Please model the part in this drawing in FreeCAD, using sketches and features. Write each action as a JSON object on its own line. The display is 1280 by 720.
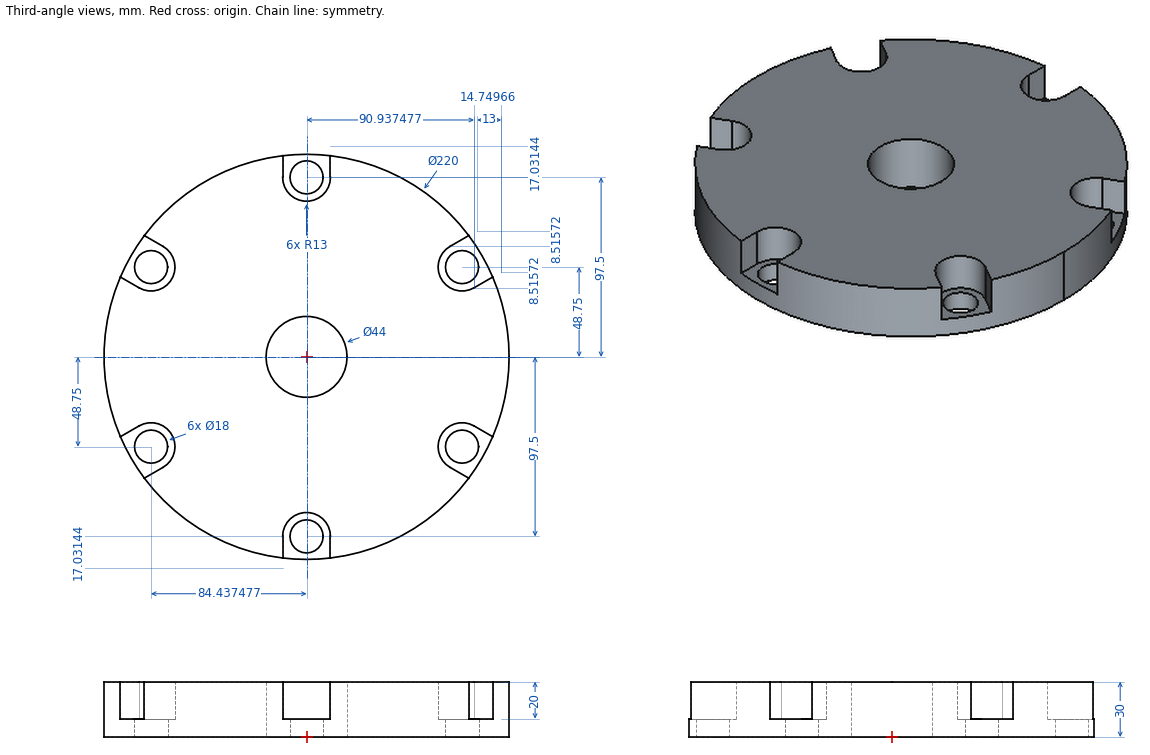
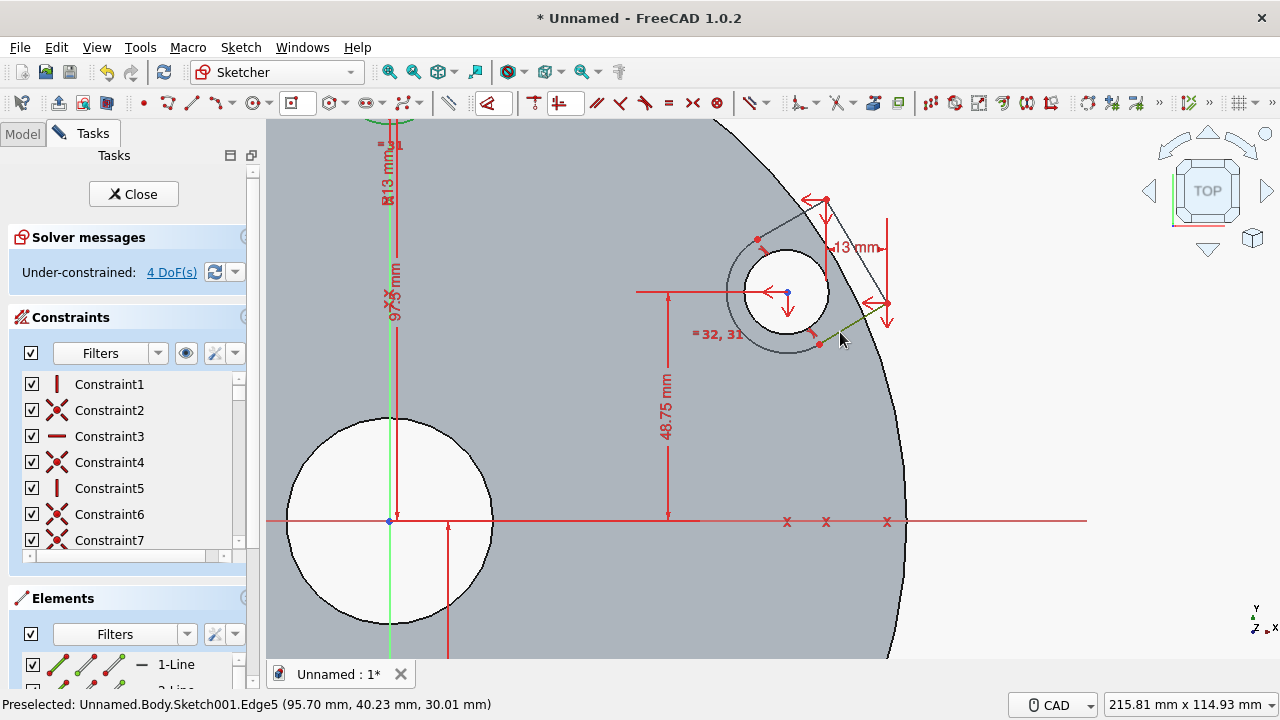
{"action": "left_click", "coordinate": [506, 104]}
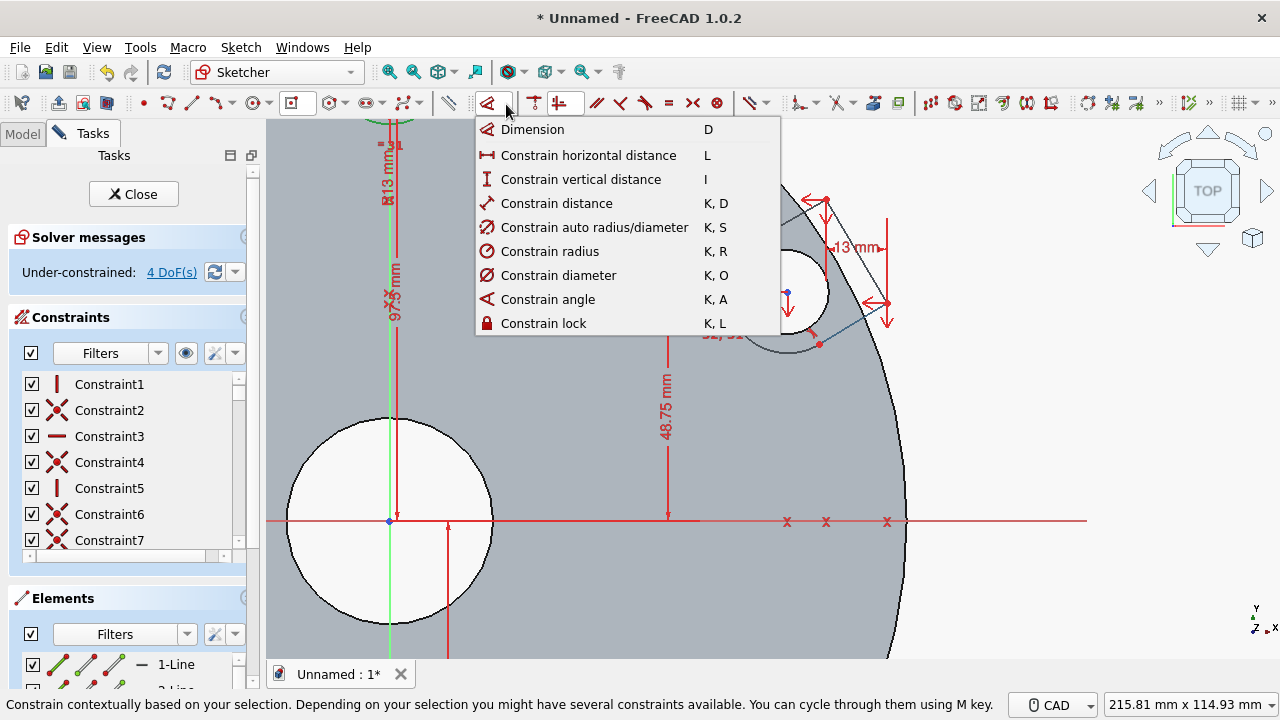
{"action": "left_click", "coordinate": [628, 179]}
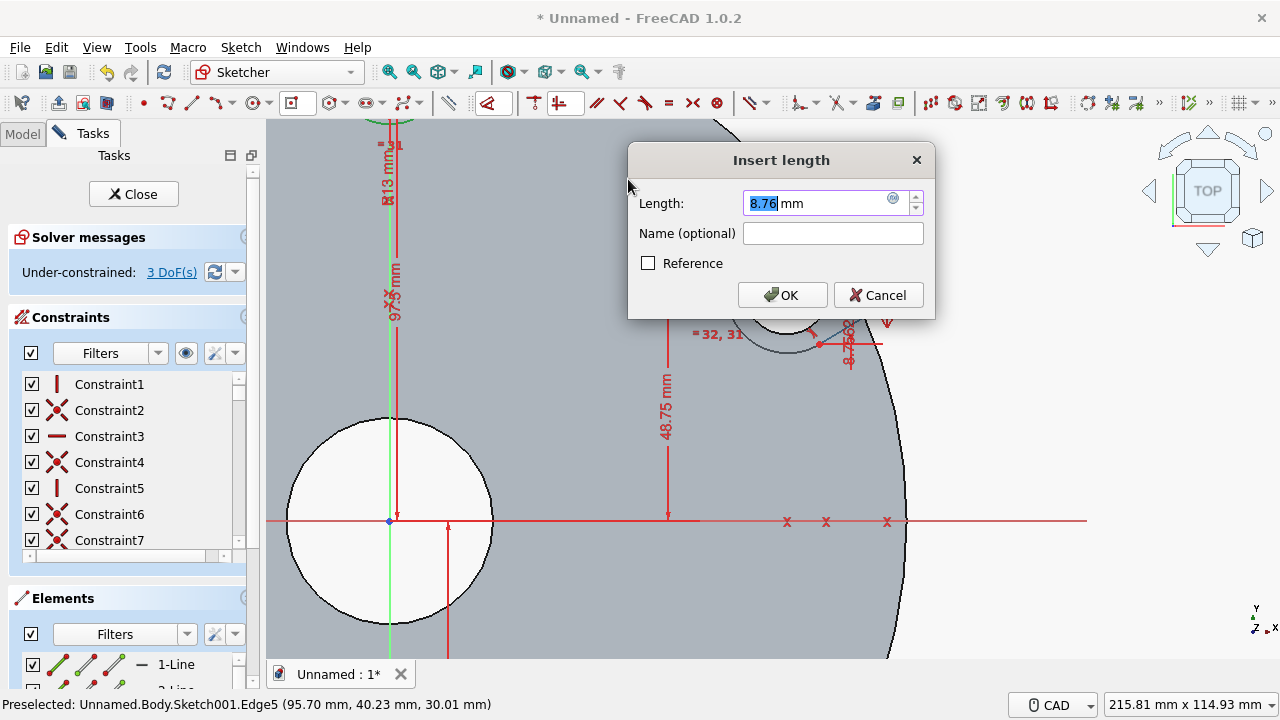
{"action": "type", "text": "8.51572"}
{"action": "key", "text": "Return"}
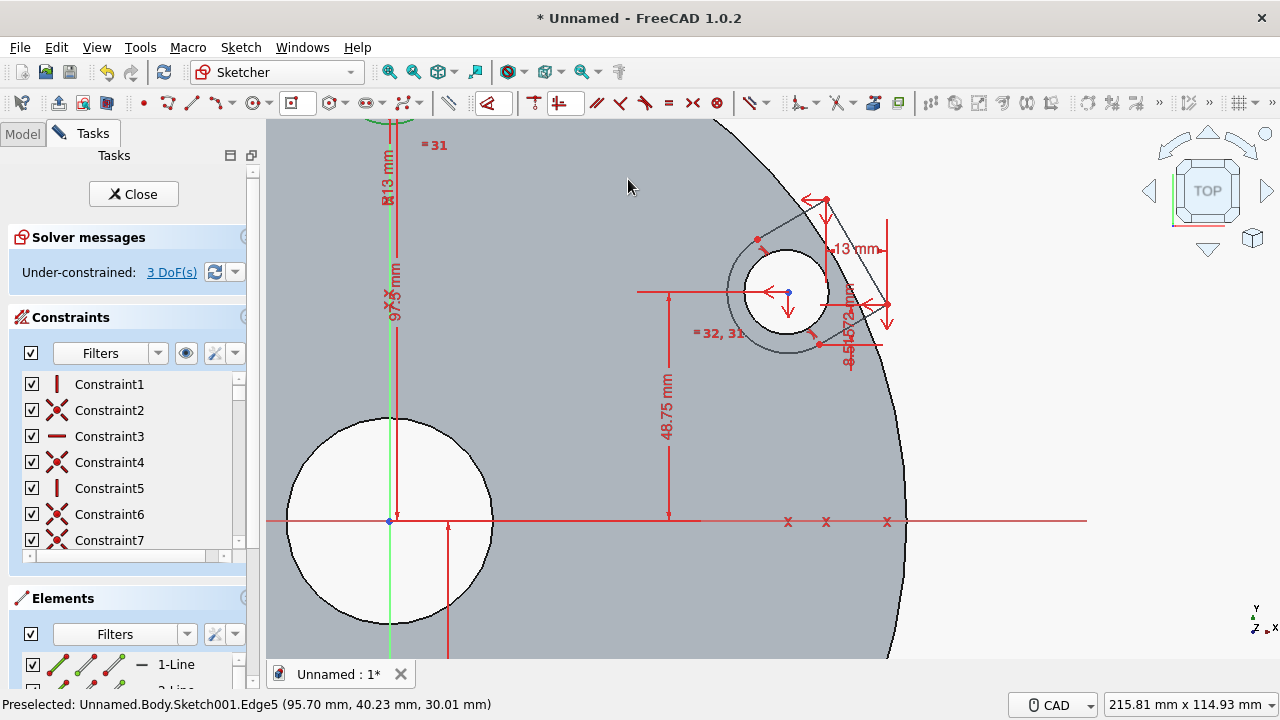
{"action": "left_click", "coordinate": [806, 212]}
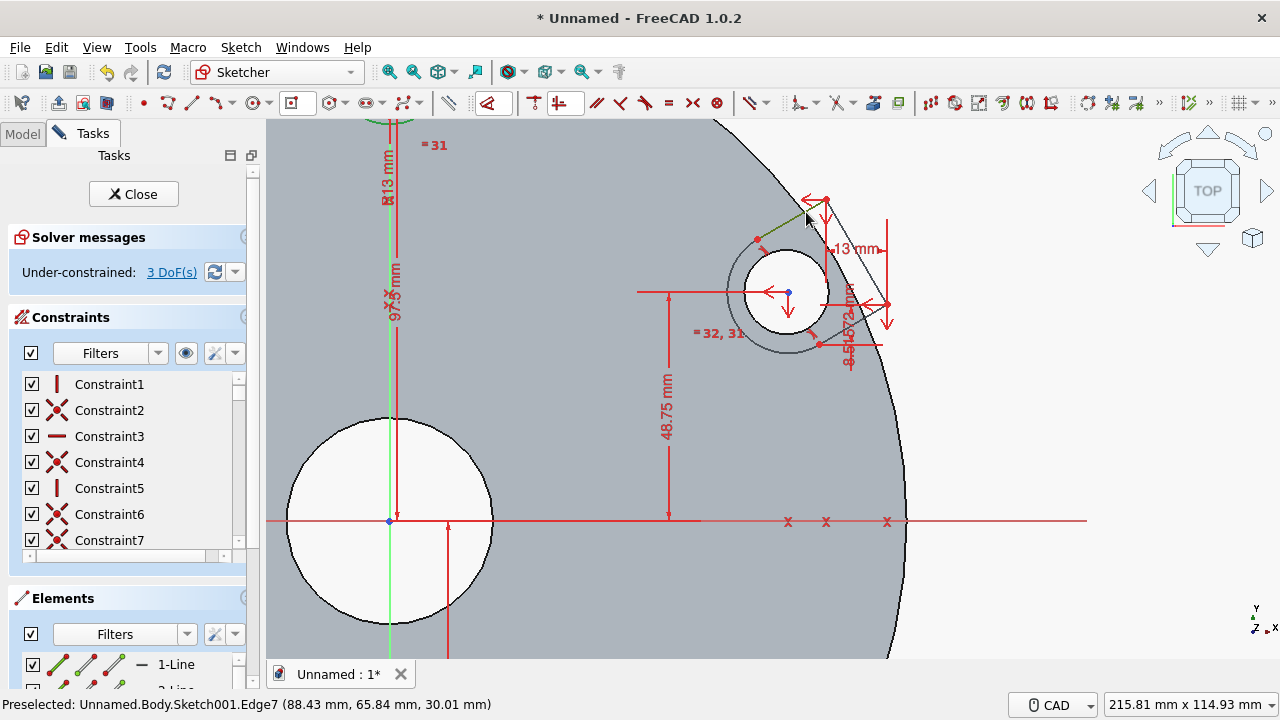
{"action": "left_click", "coordinate": [506, 104]}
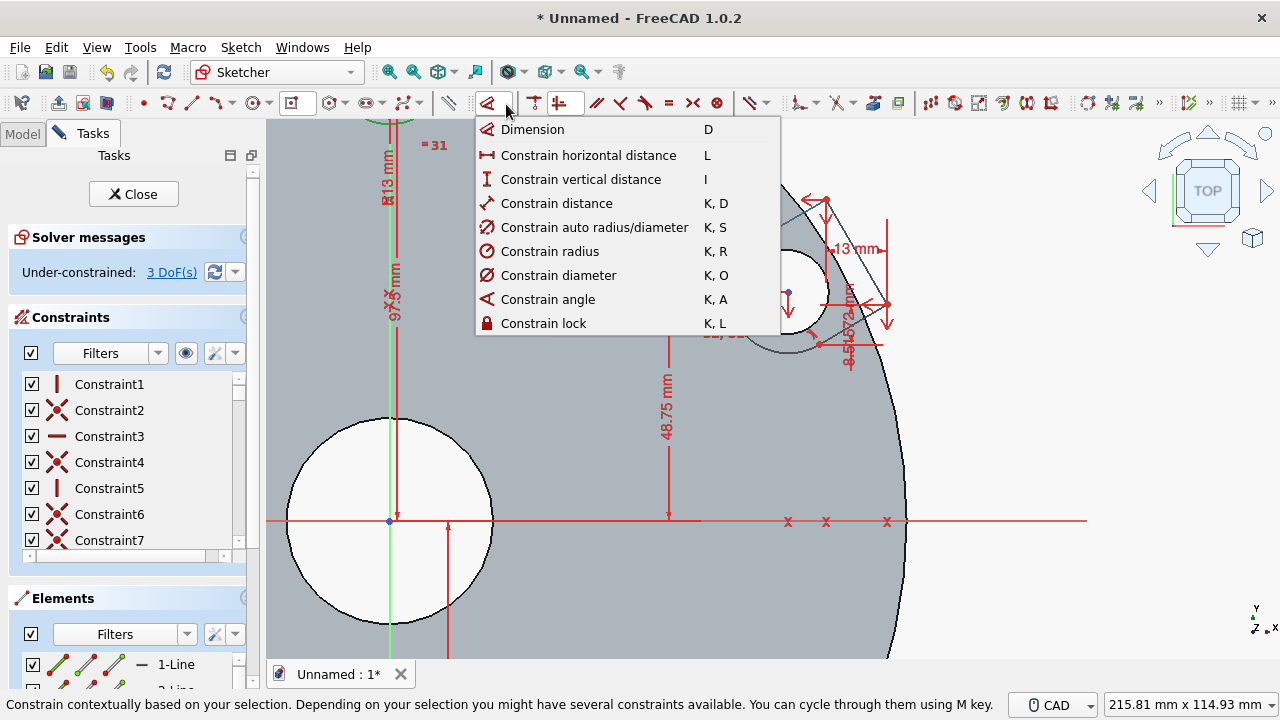
{"action": "left_click", "coordinate": [628, 179]}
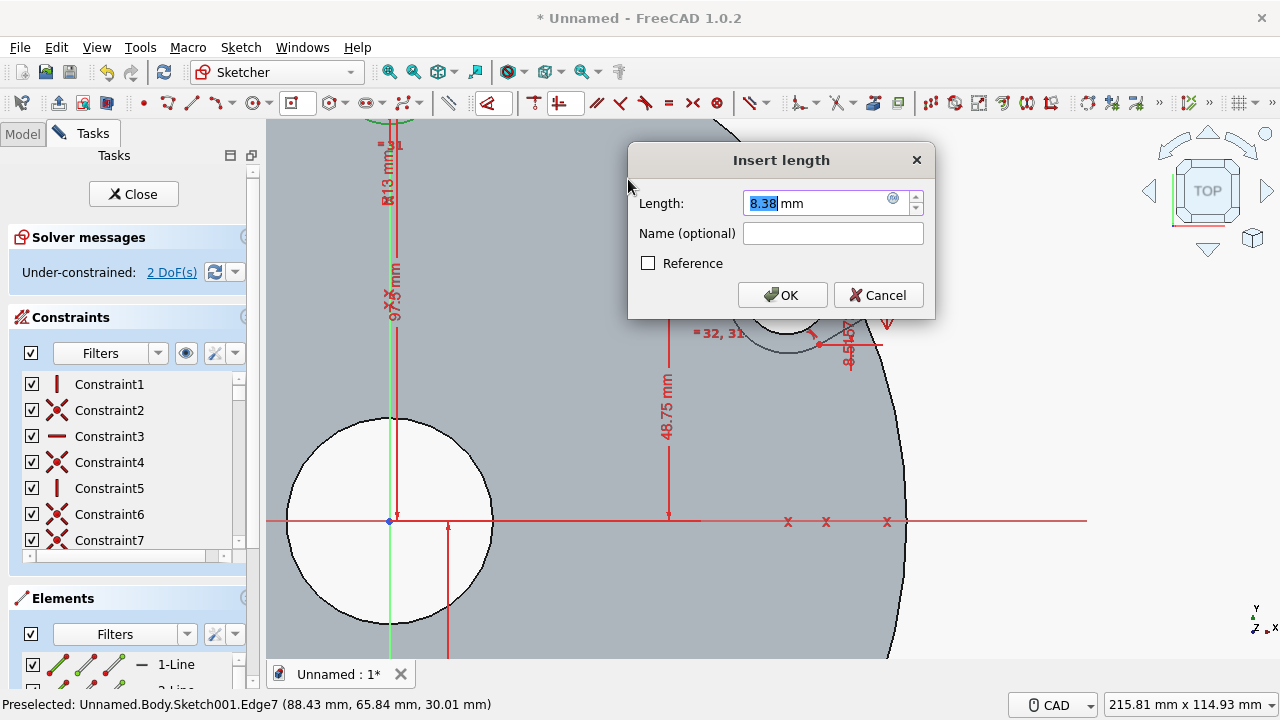
{"action": "type", "text": "8.51572"}
{"action": "key", "text": "Return"}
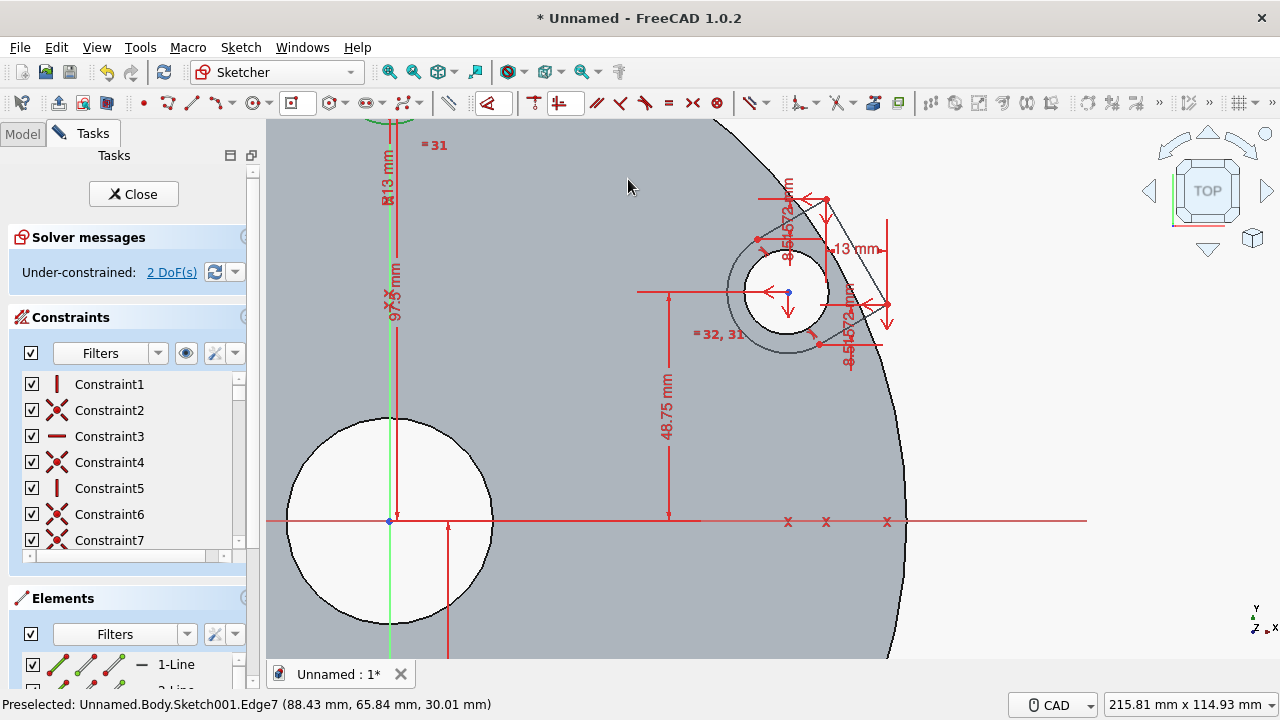
{"action": "left_click", "coordinate": [840, 333]}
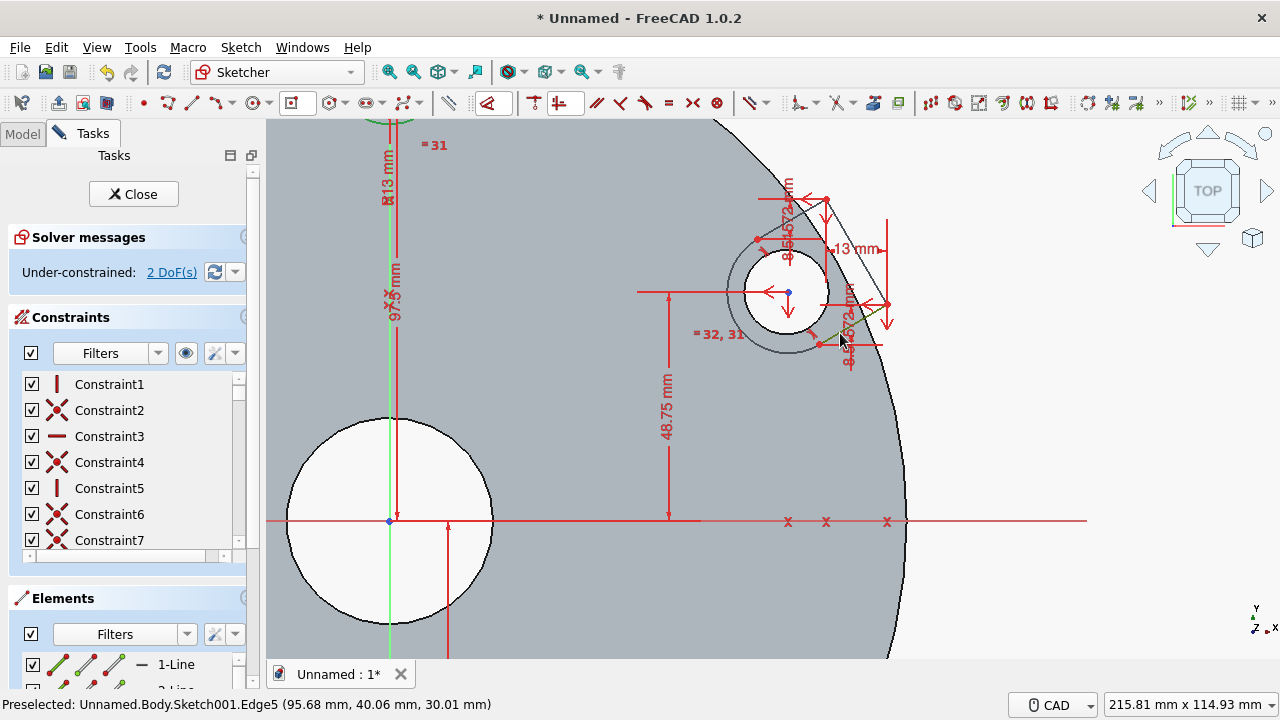
{"action": "left_click", "coordinate": [506, 104]}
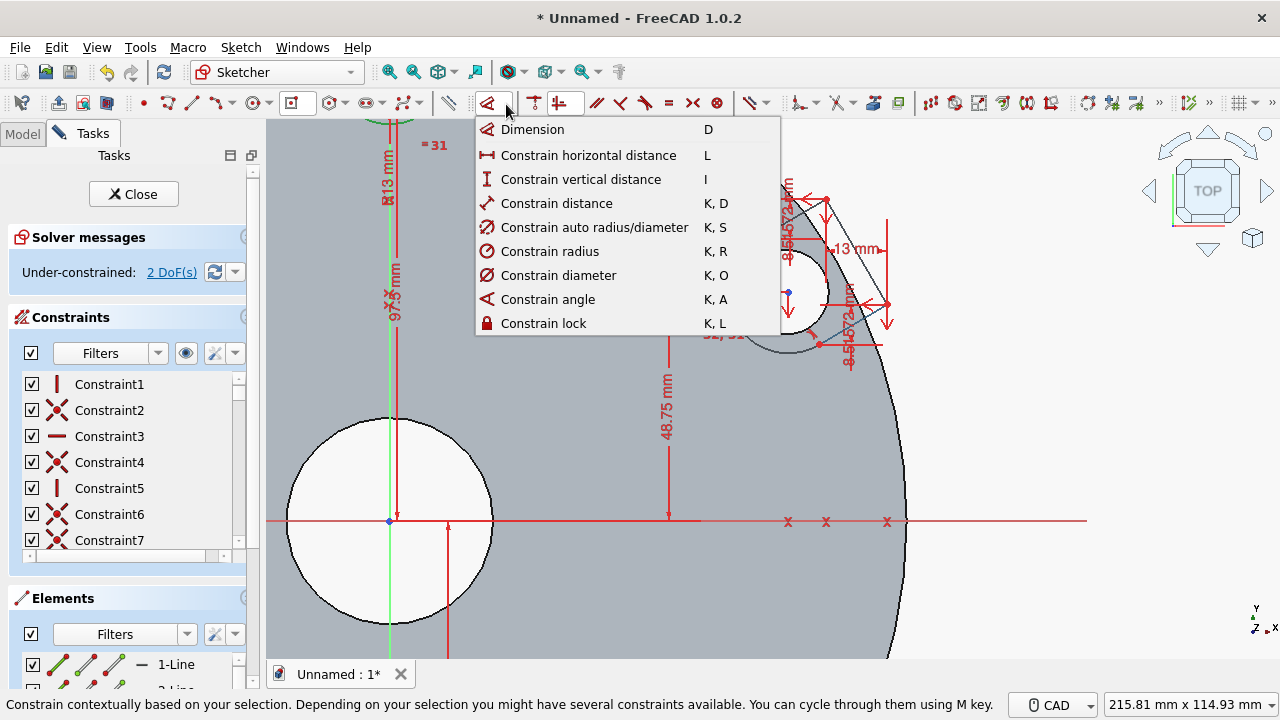
{"action": "left_click", "coordinate": [628, 155]}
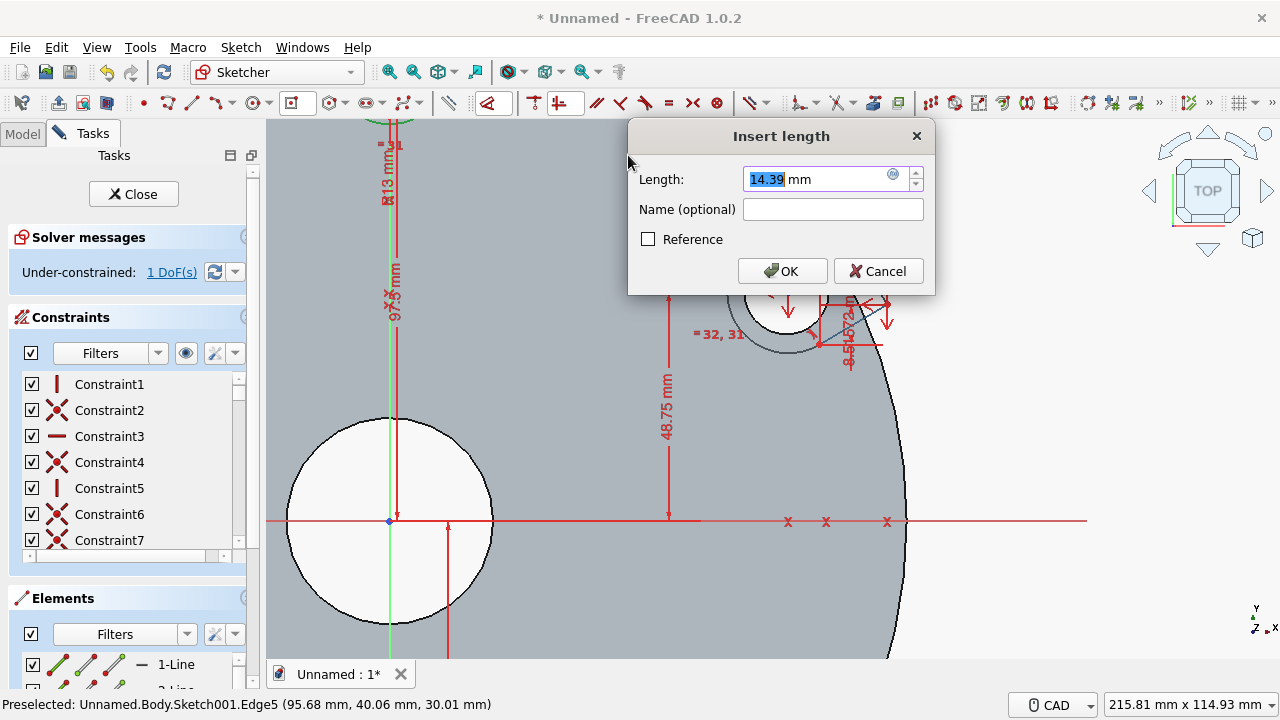
{"action": "type", "text": "14.74966"}
{"action": "key", "text": "Return"}